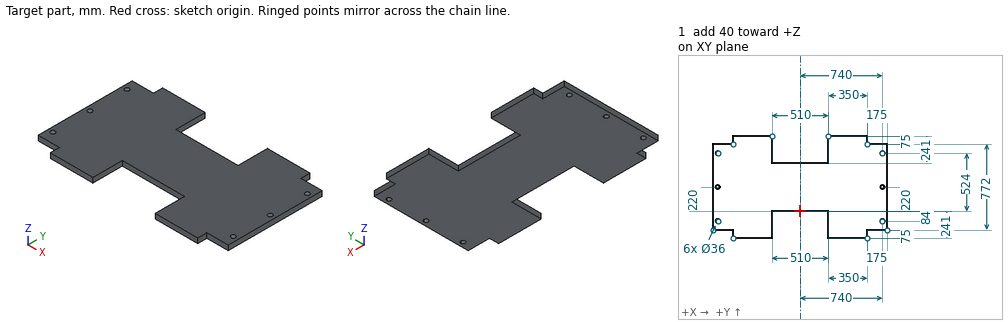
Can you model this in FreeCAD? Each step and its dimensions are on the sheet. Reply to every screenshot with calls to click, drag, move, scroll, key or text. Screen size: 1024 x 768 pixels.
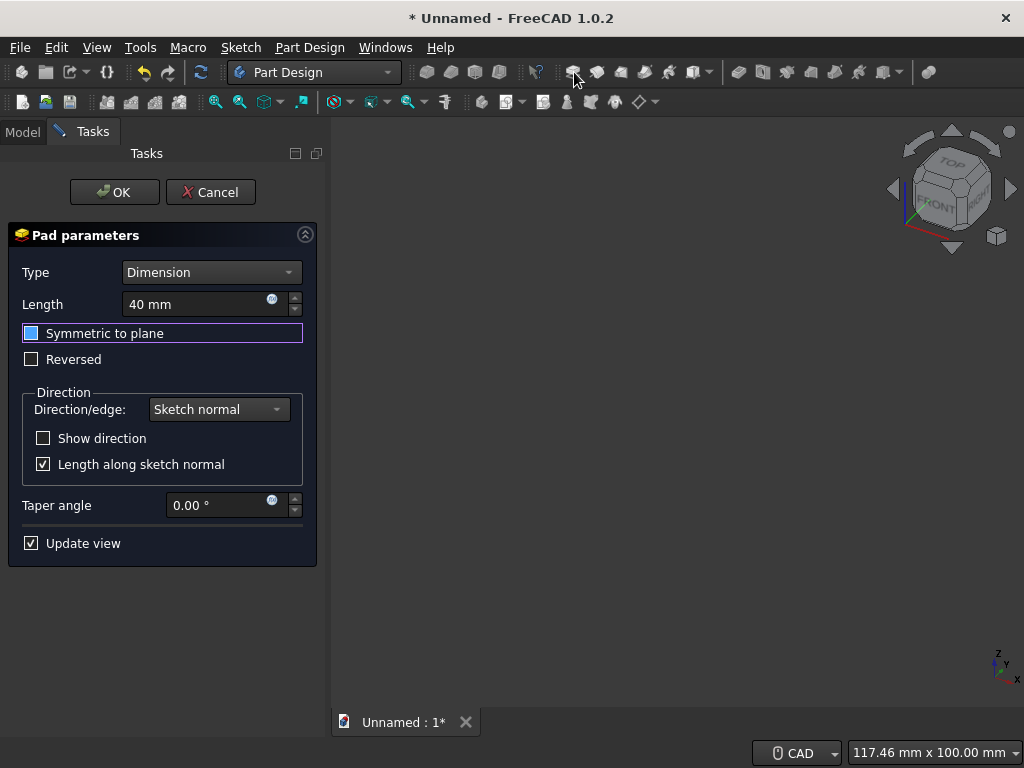
click(115, 192)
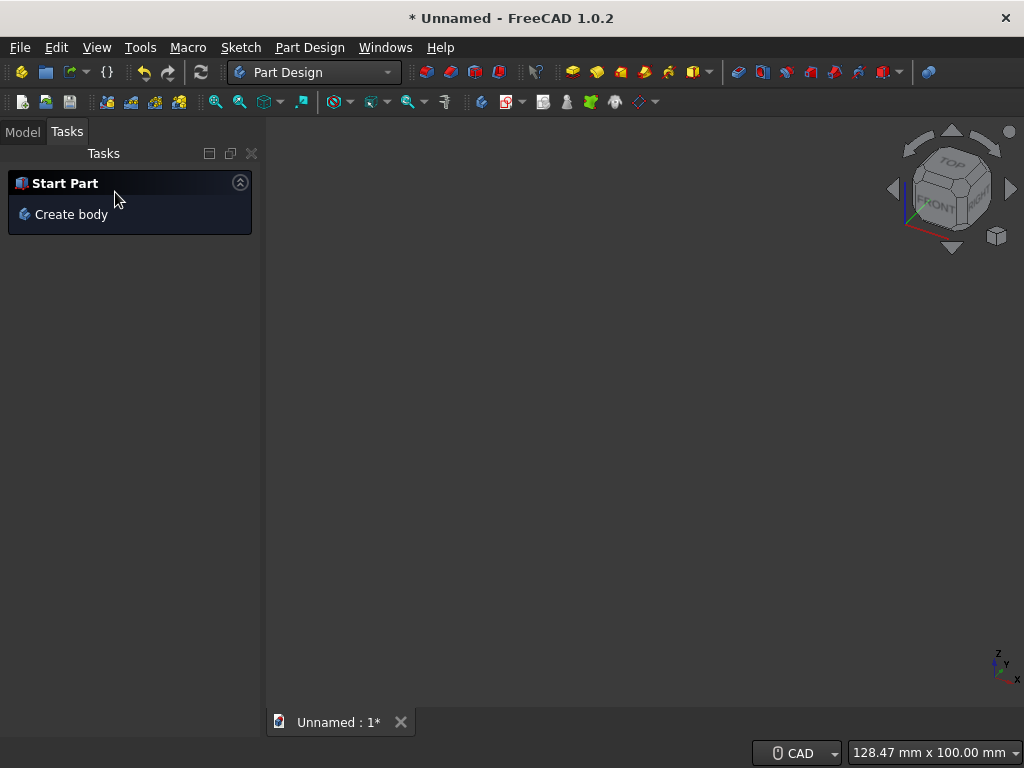
key(0)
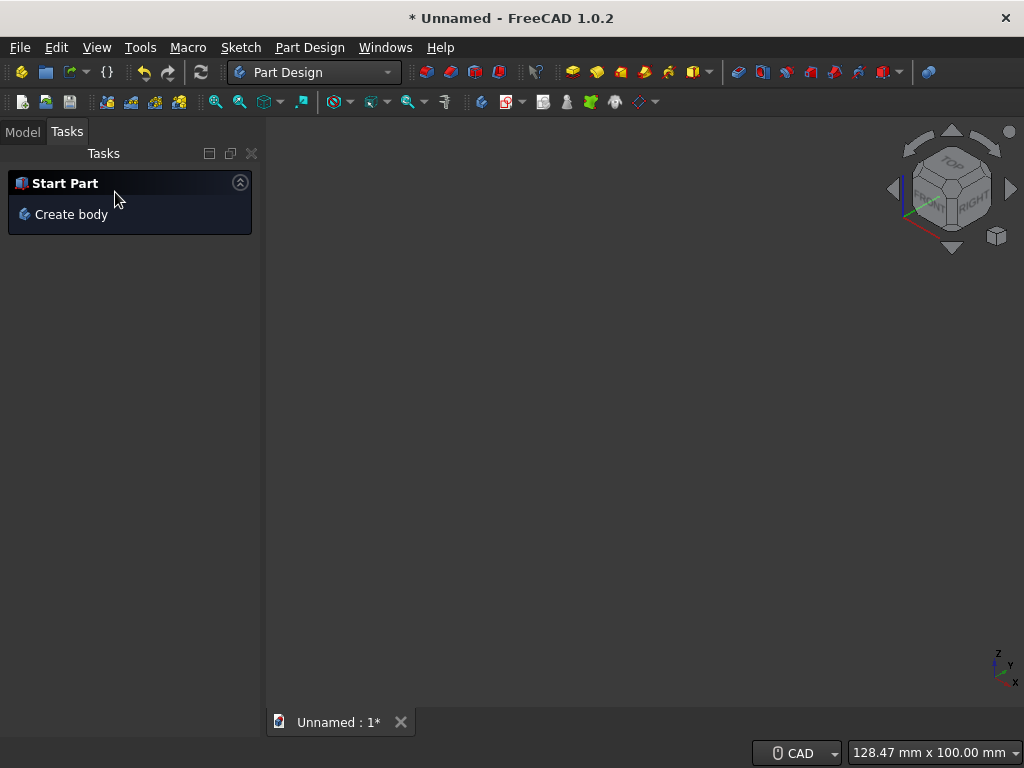
click(216, 102)